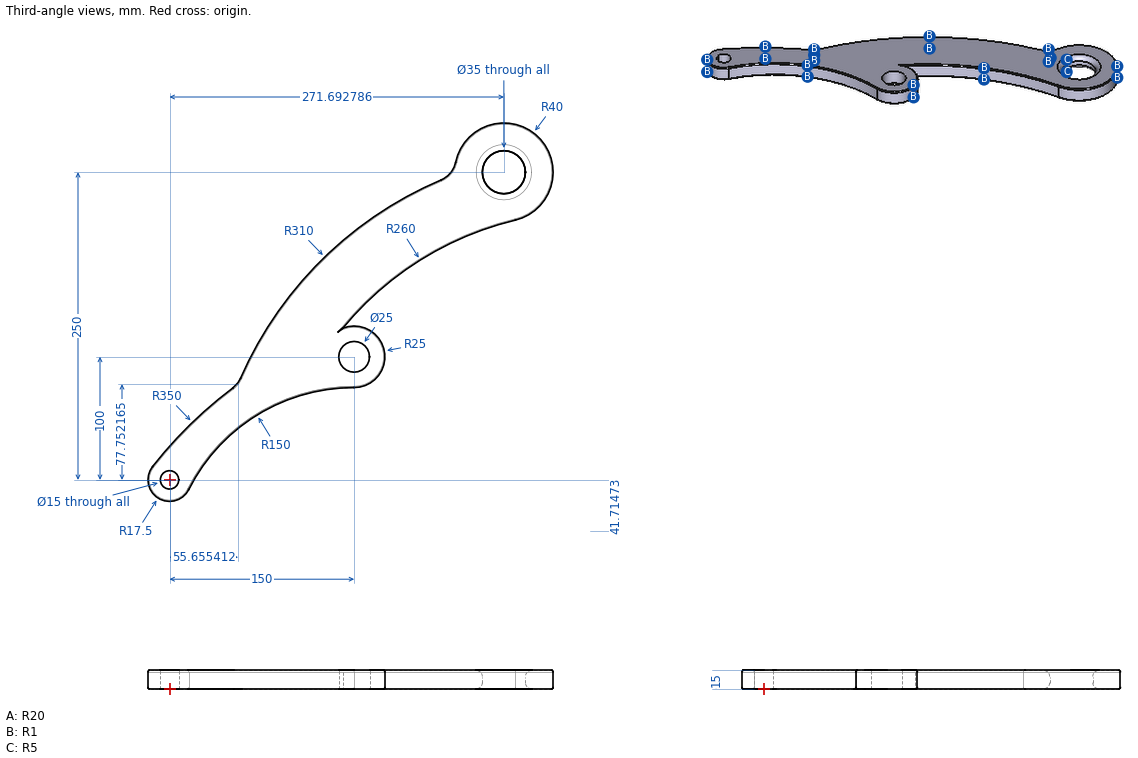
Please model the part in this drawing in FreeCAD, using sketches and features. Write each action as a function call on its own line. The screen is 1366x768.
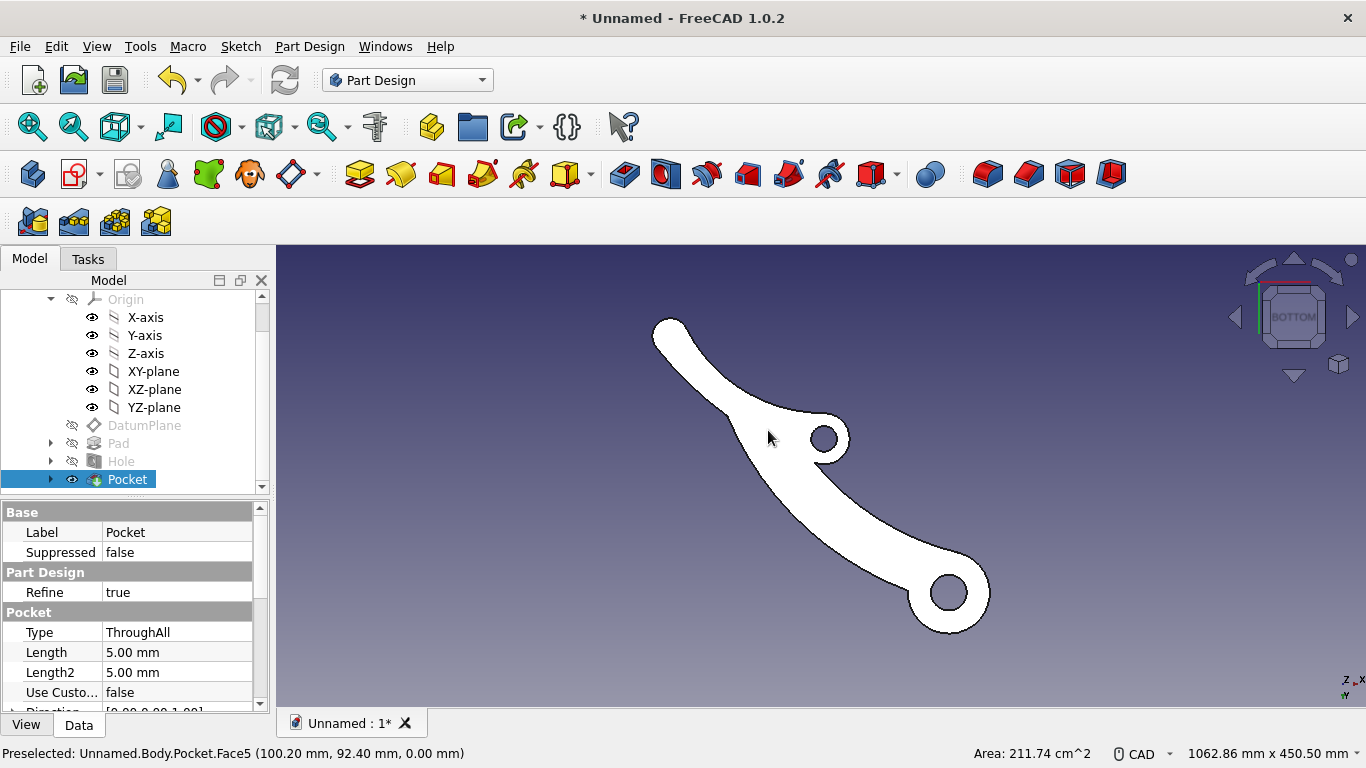
click(74, 174)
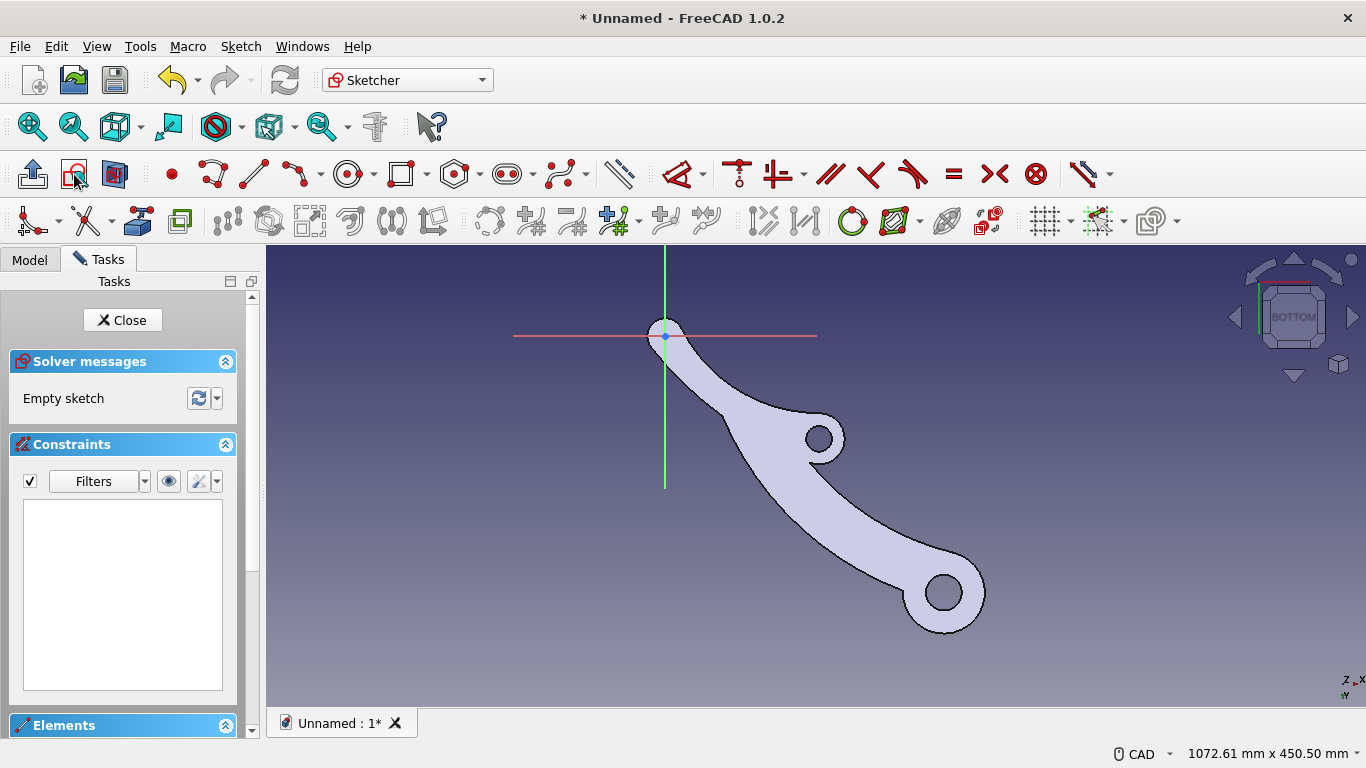
scroll(661, 329, up, 15)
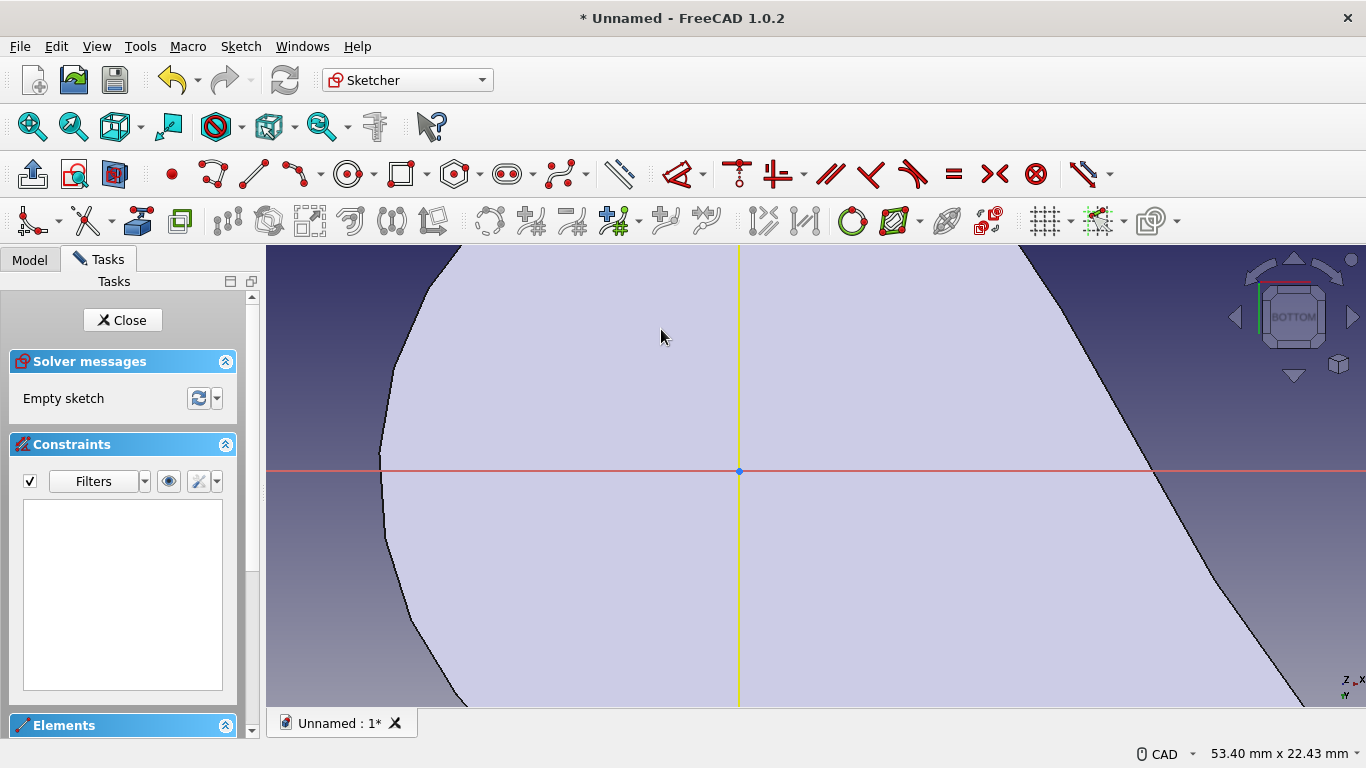
click(348, 174)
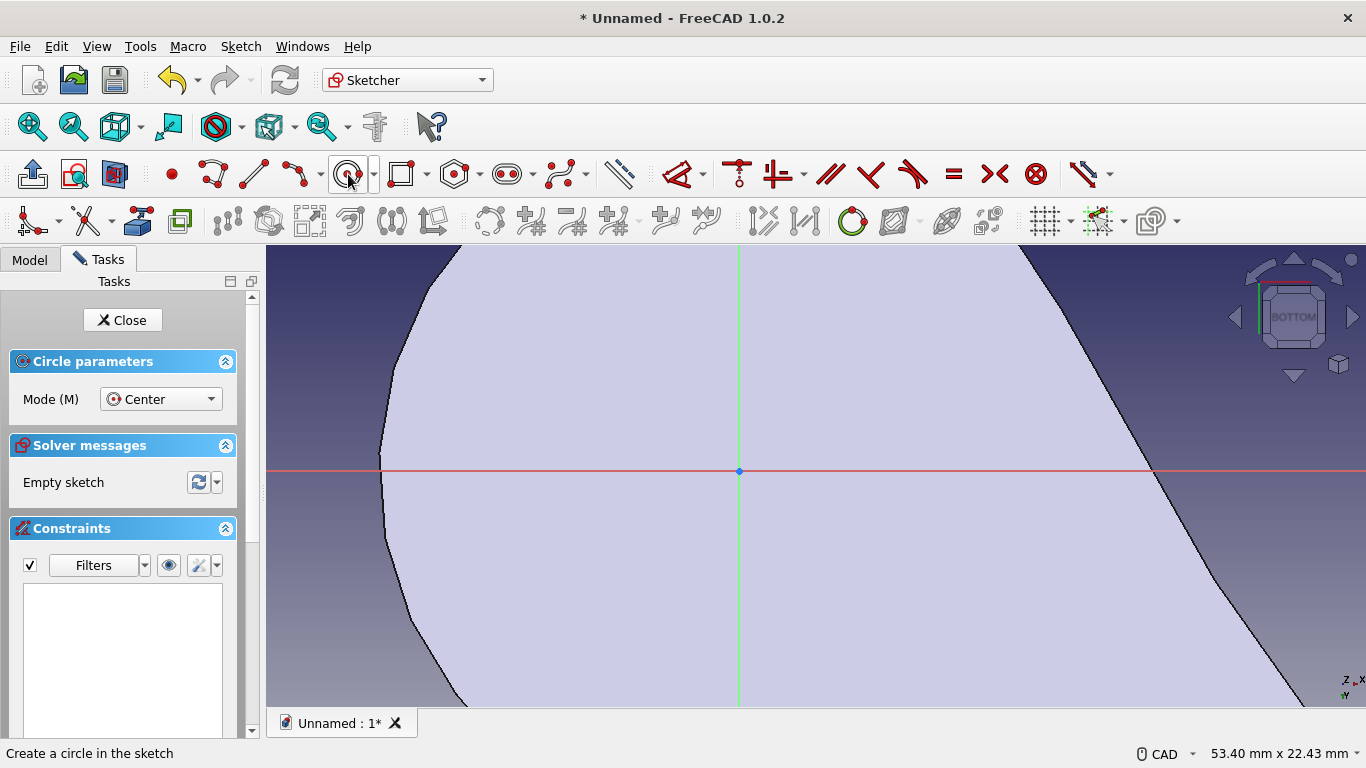
click(739, 471)
move(849, 362)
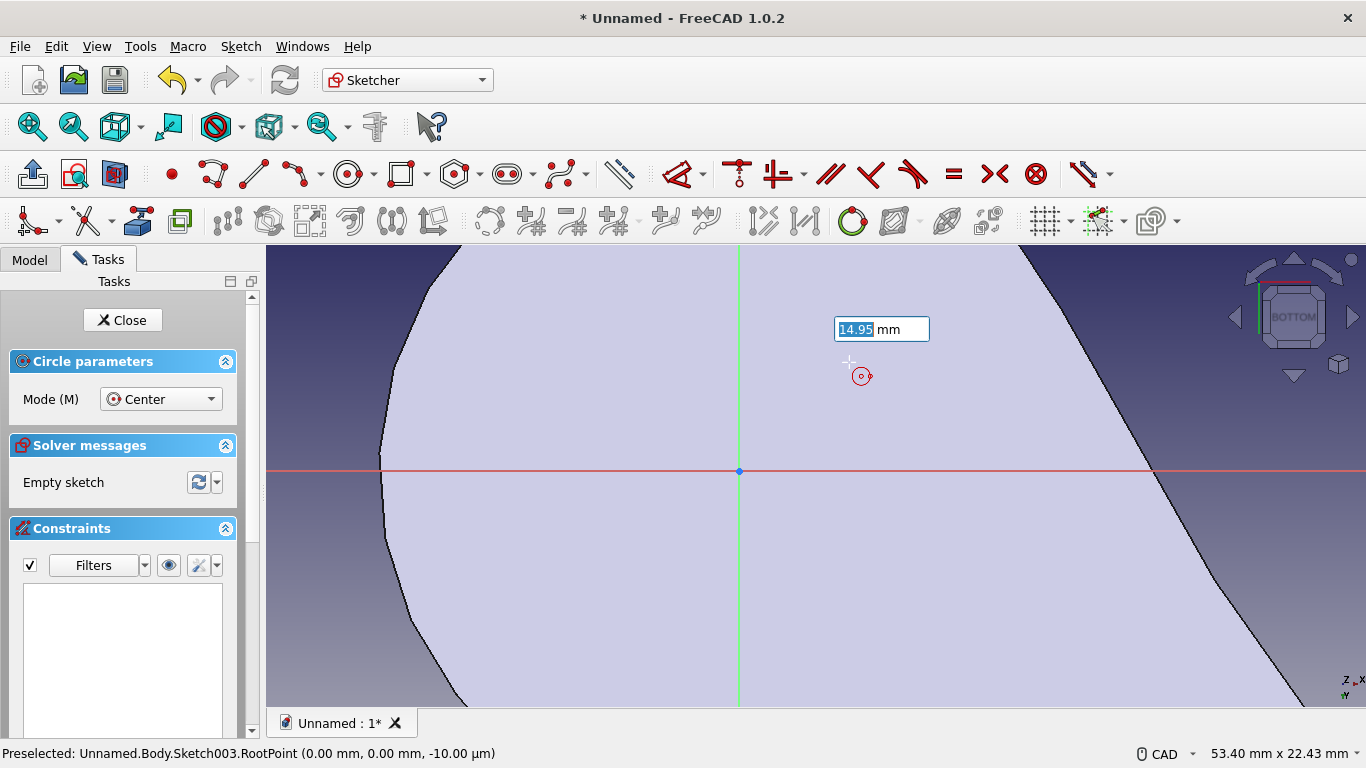
text(15)
key(Return)
key(Escape)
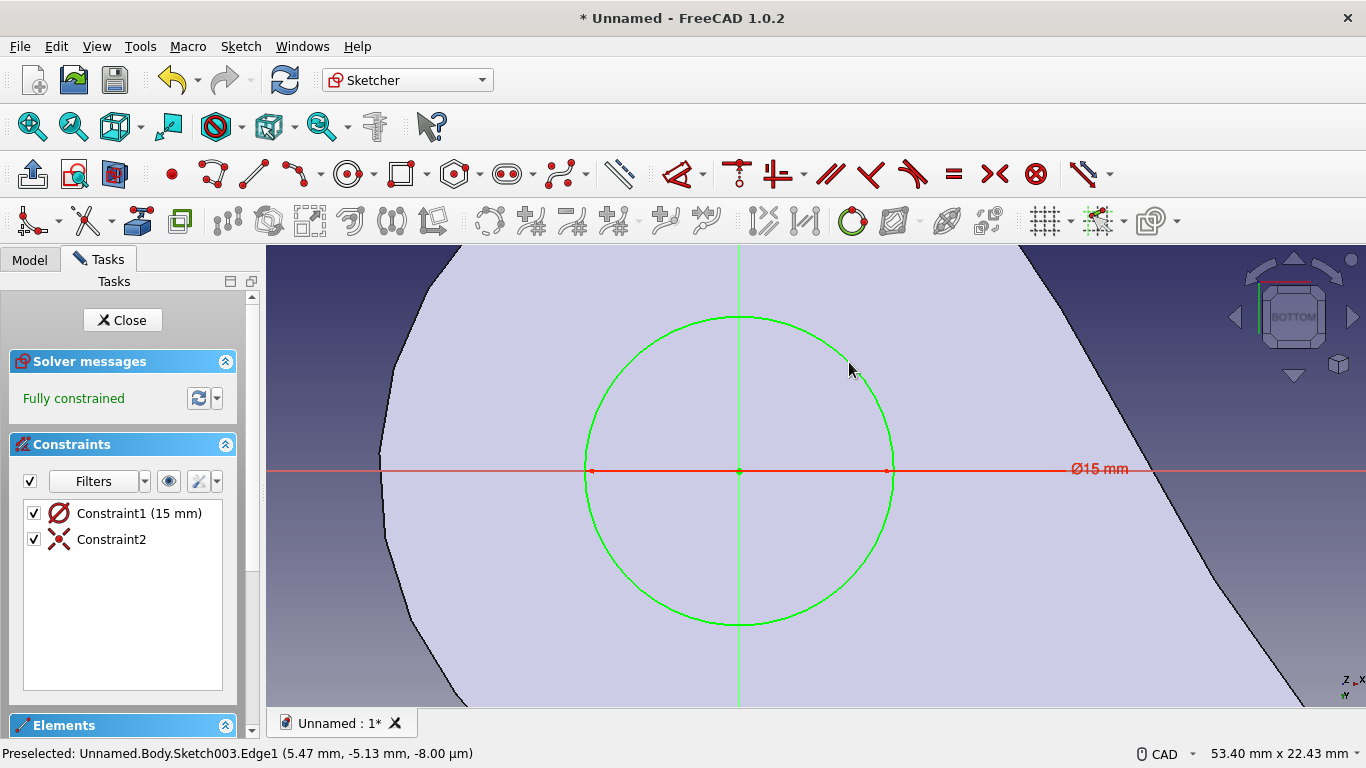
click(123, 320)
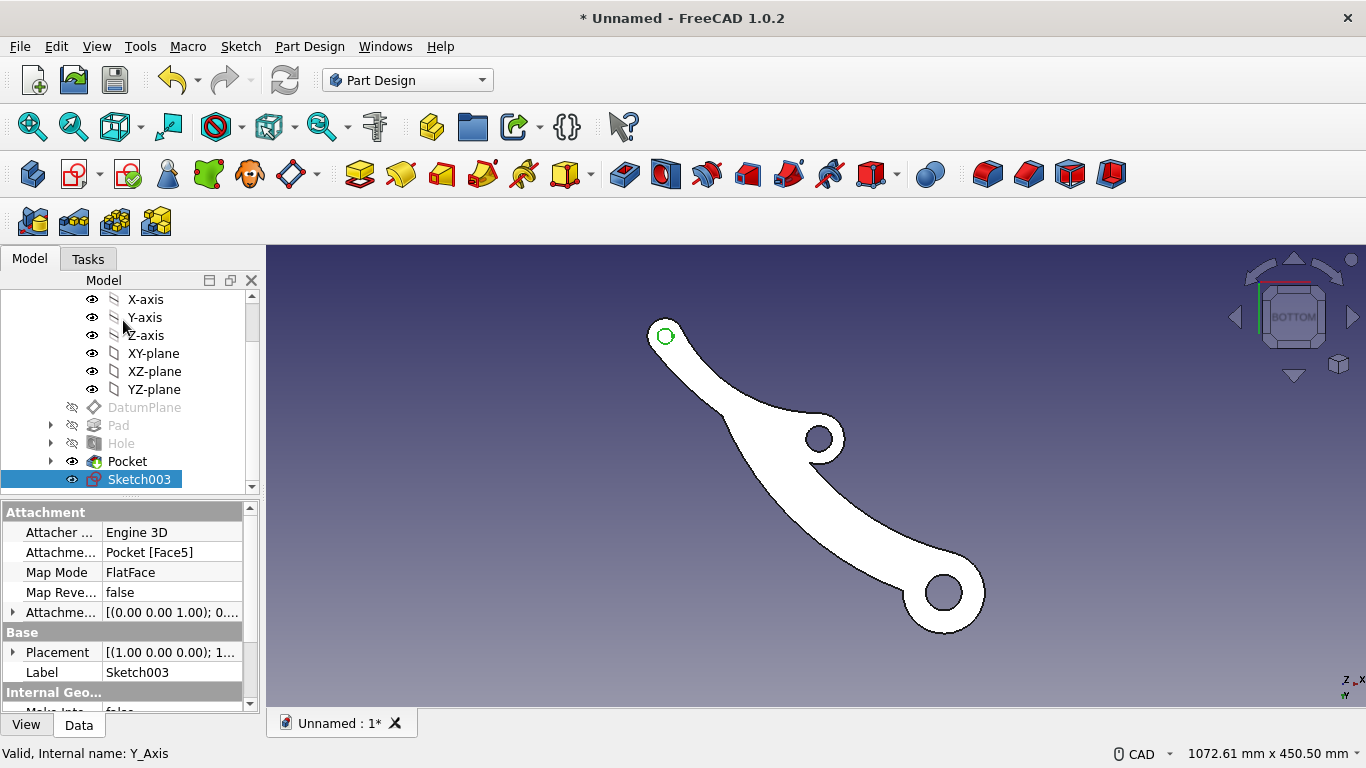
click(666, 174)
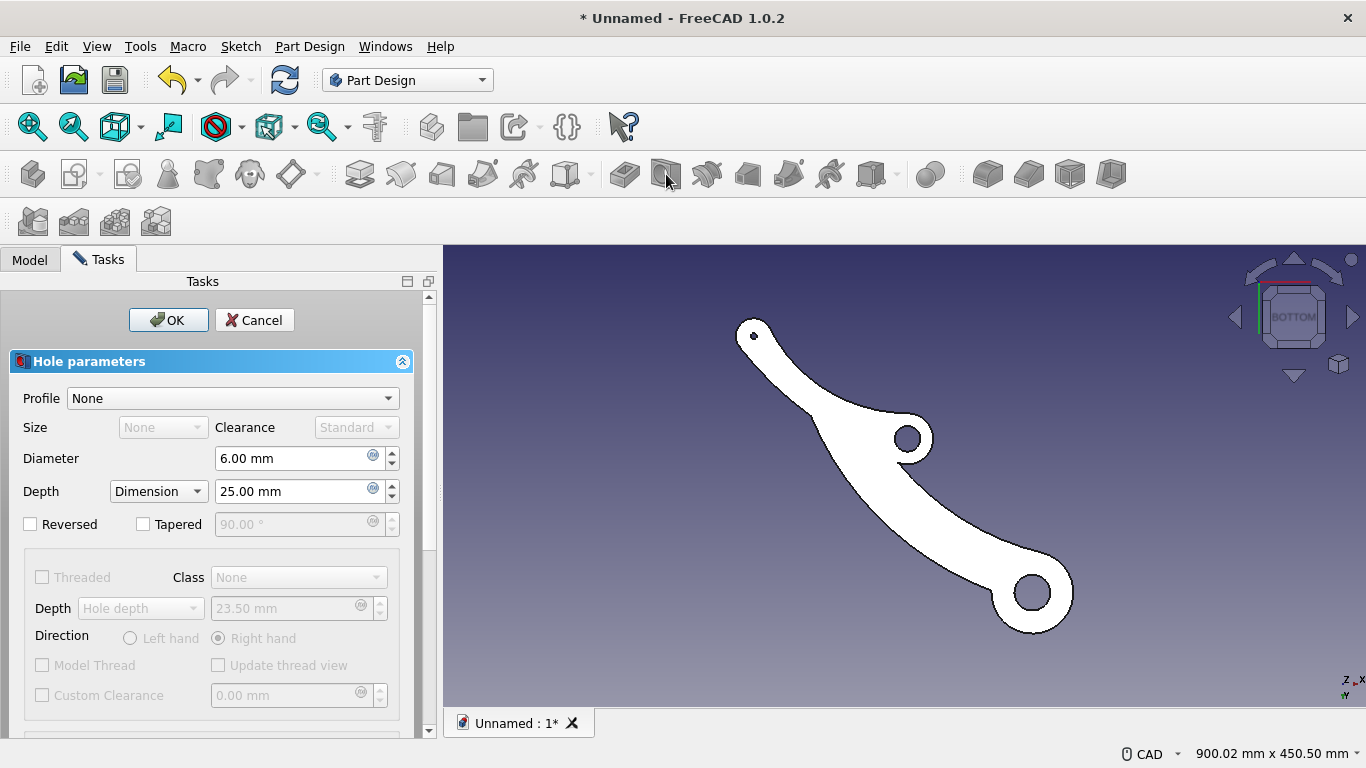
triple_click(300, 458)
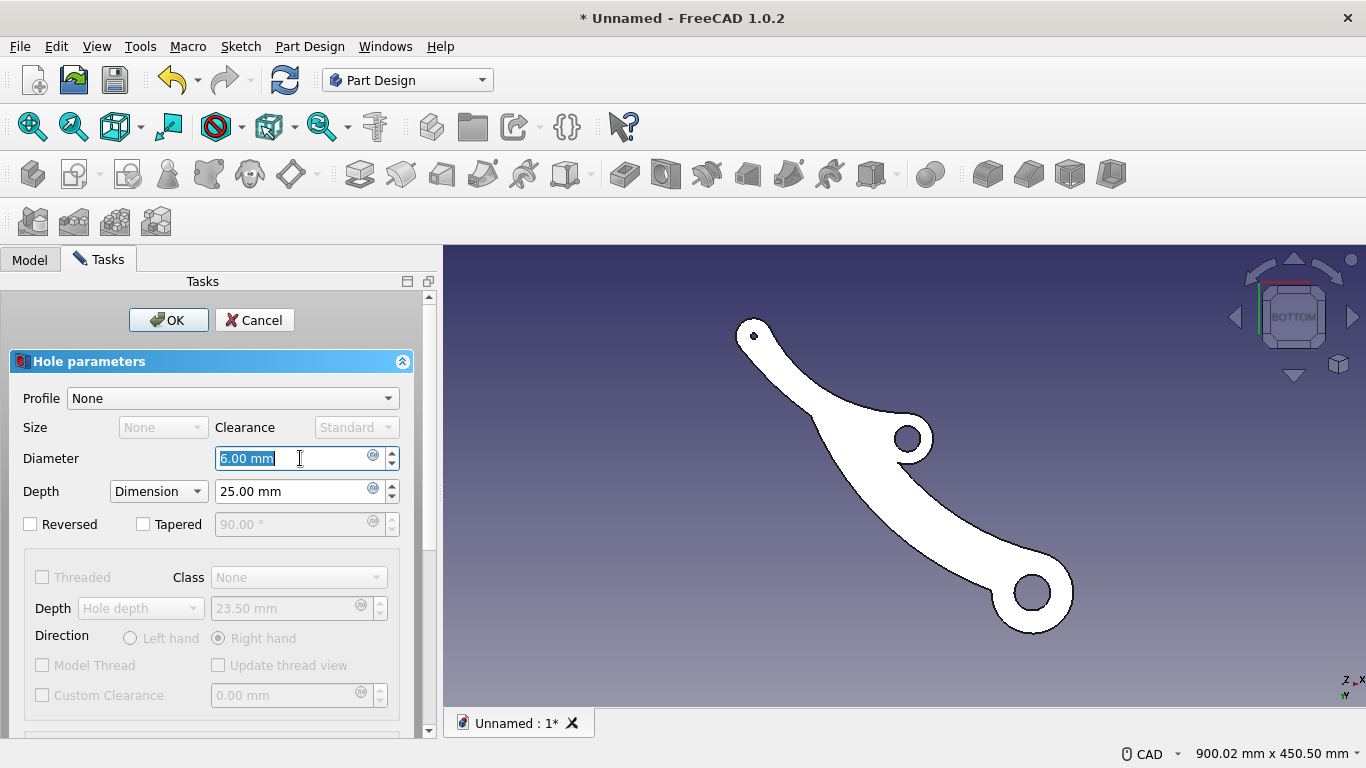
text(15)
key(Tab)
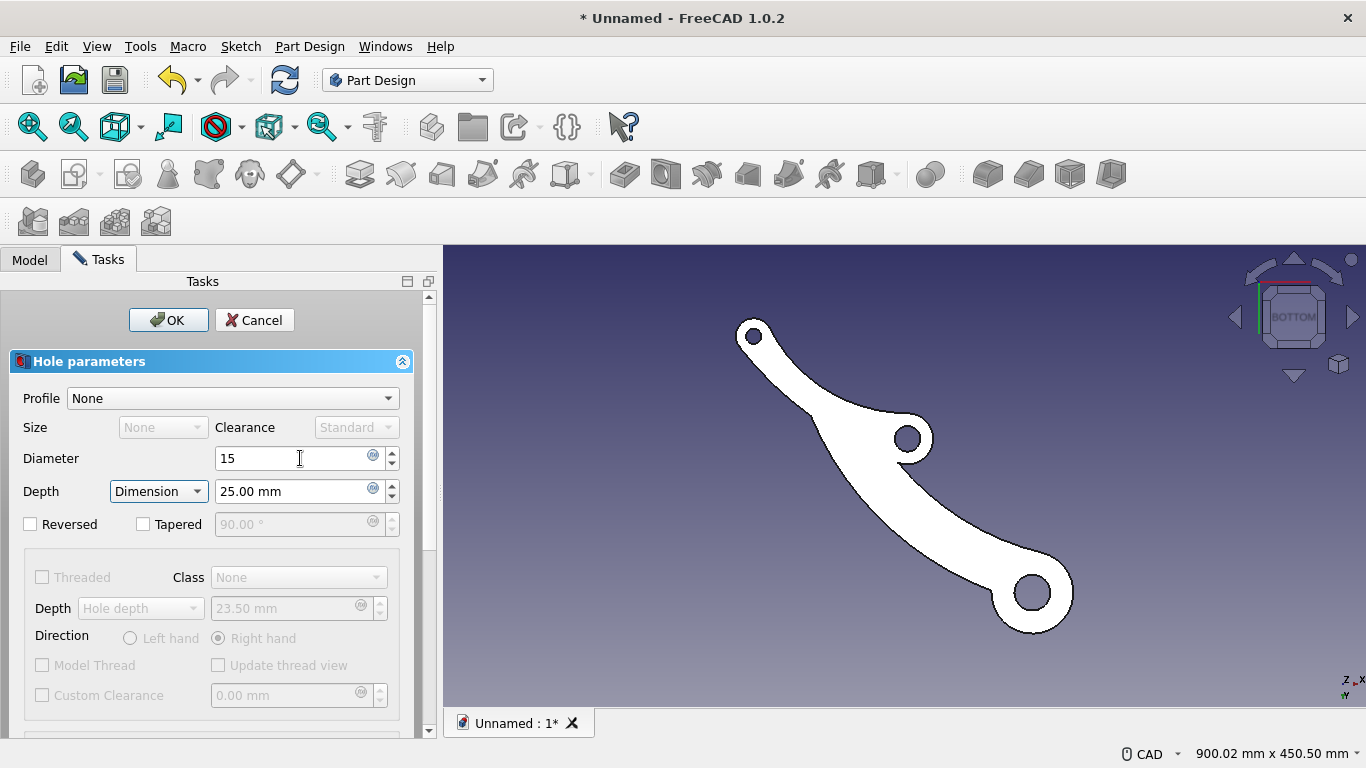
click(160, 492)